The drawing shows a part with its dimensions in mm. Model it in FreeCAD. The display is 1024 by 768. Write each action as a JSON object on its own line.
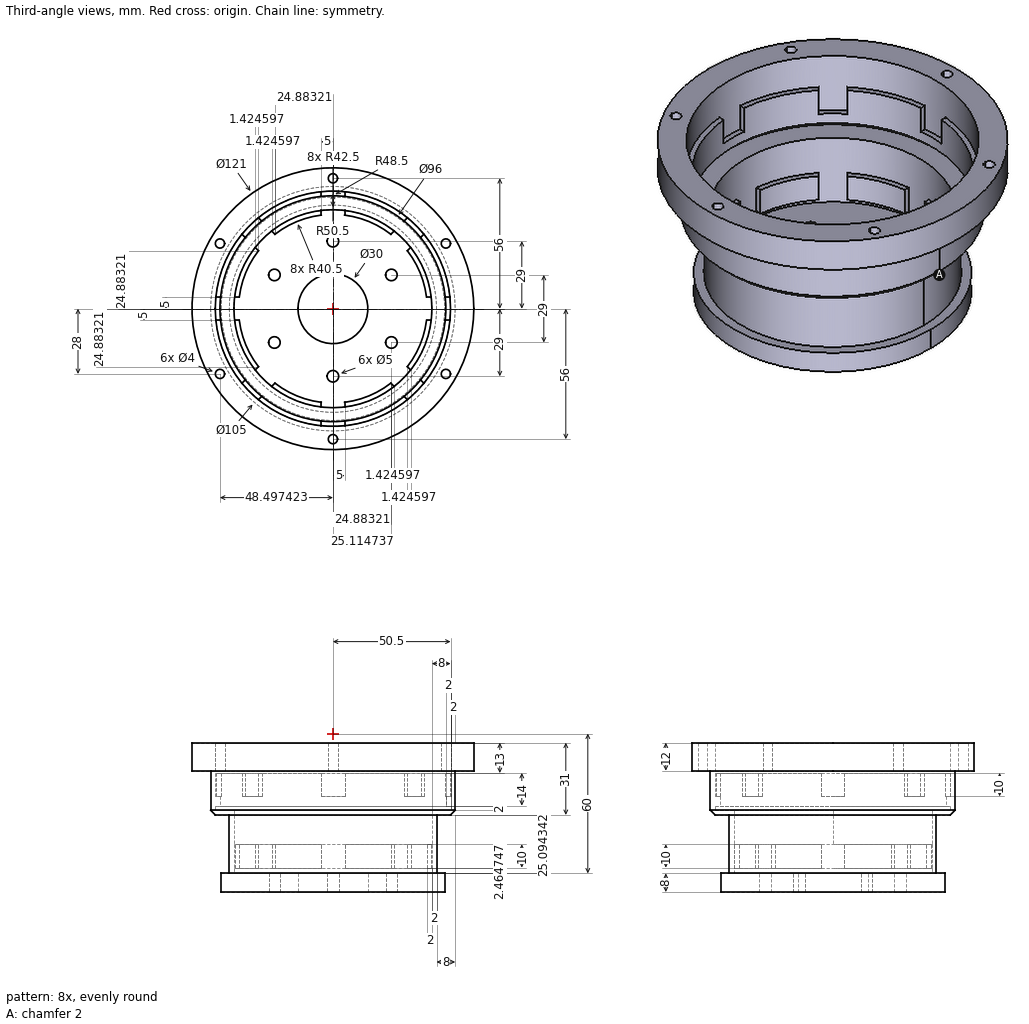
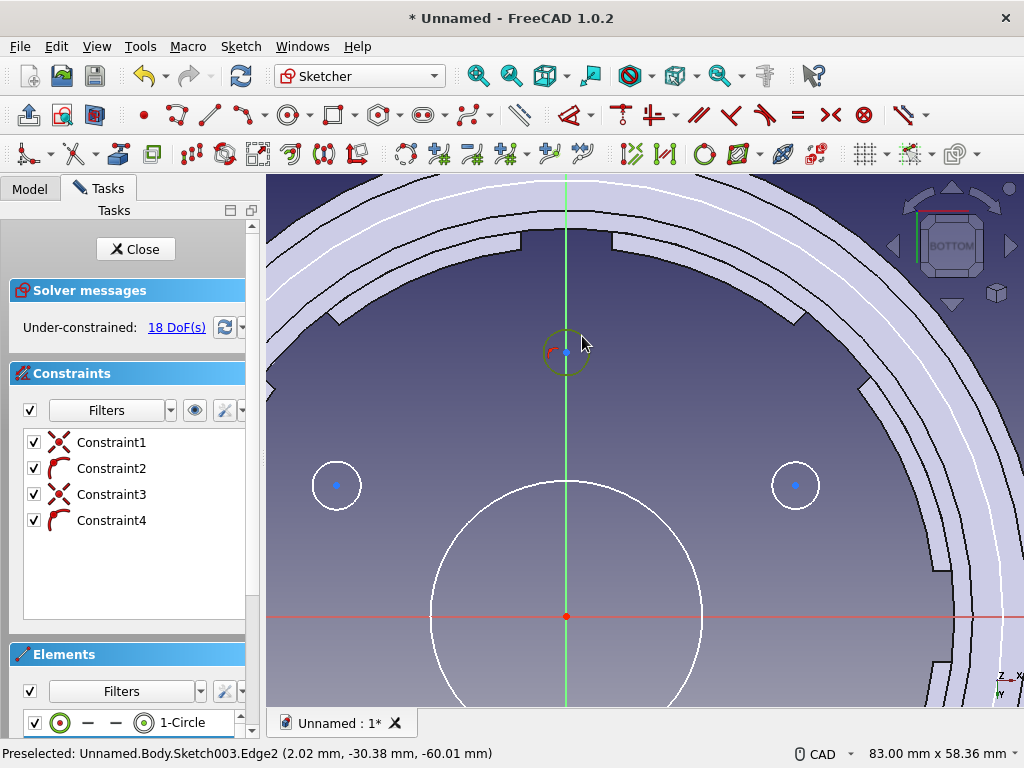
{"action": "left_click", "coordinate": [812, 469]}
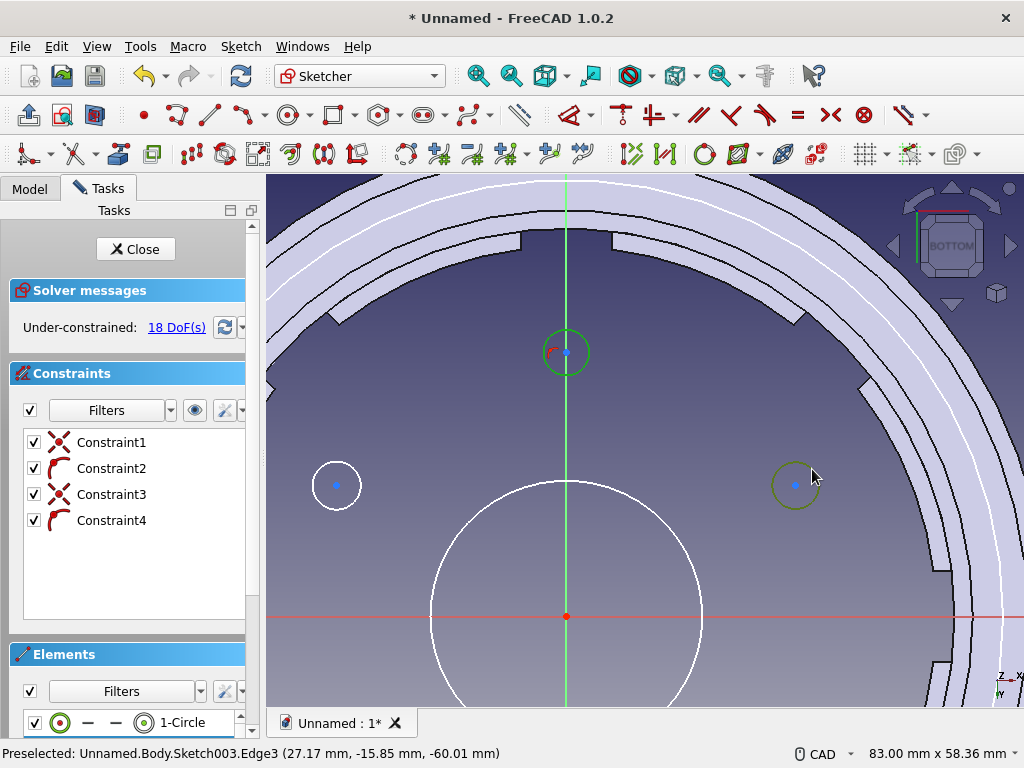
{"action": "left_click", "coordinate": [354, 469]}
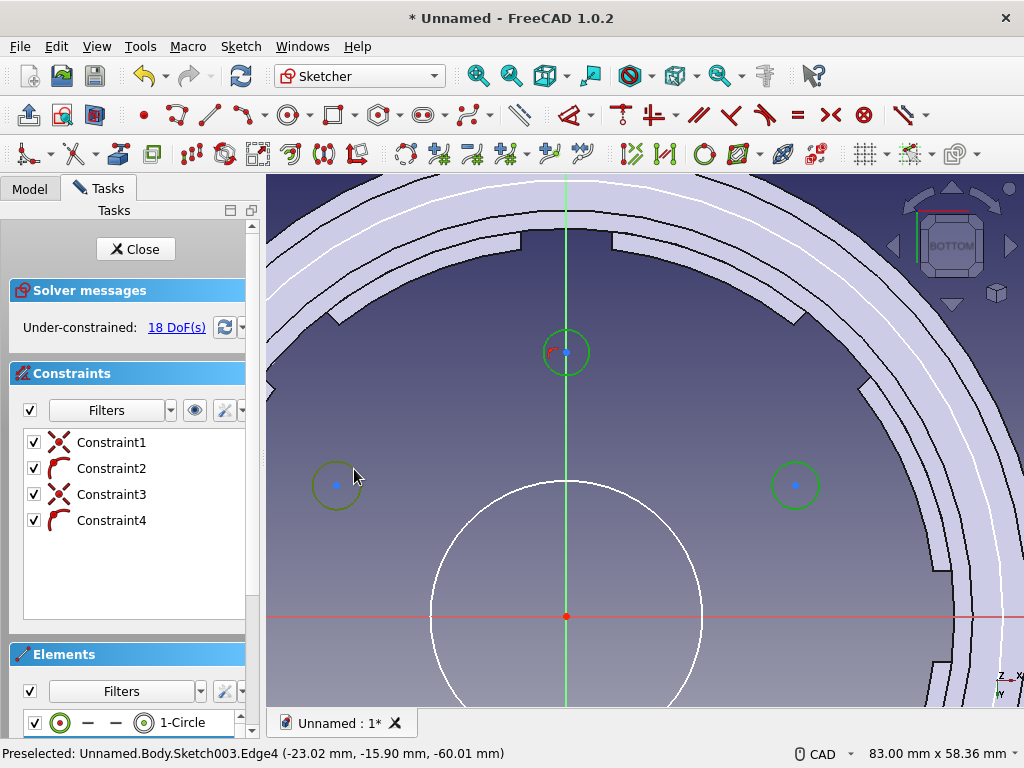
{"action": "scroll", "coordinate": [582, 338], "scroll_direction": "down", "scroll_amount": 5}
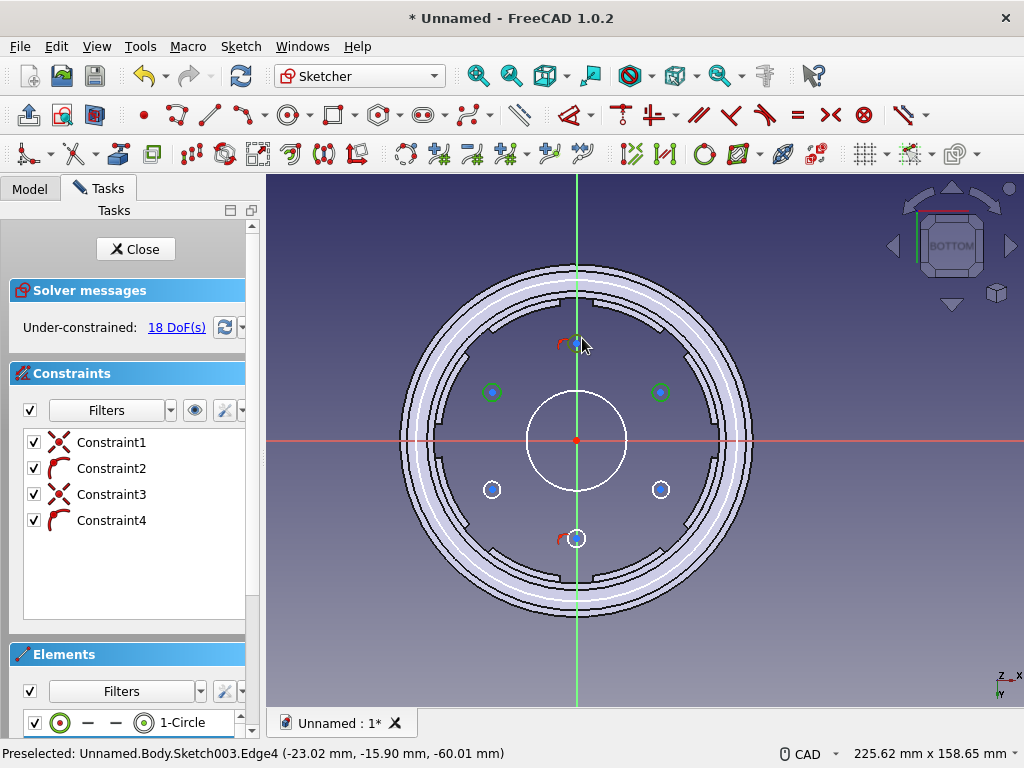
{"action": "scroll", "coordinate": [667, 484], "scroll_direction": "up", "scroll_amount": 3}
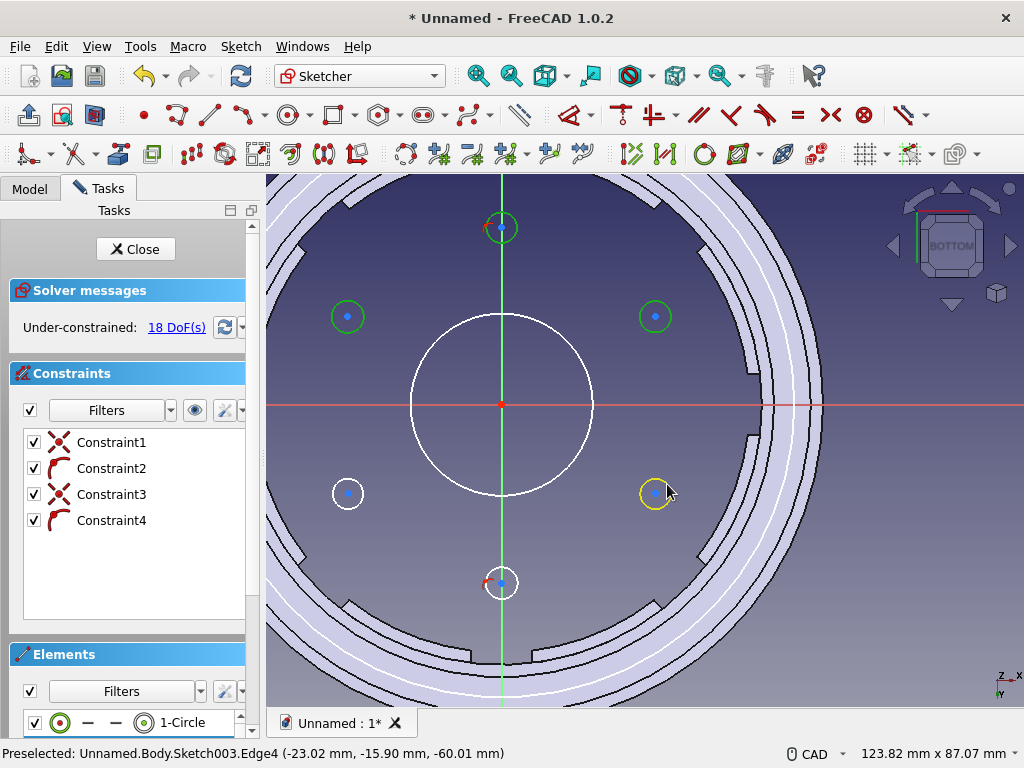
{"action": "left_click", "coordinate": [666, 483]}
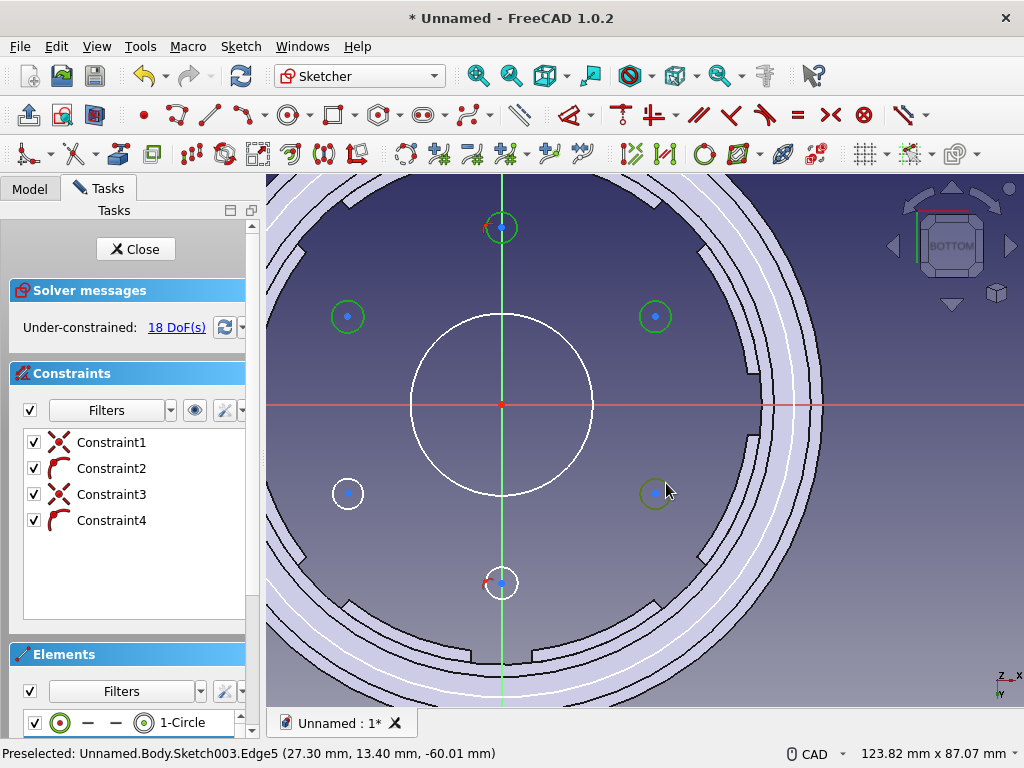
{"action": "scroll", "coordinate": [513, 572], "scroll_direction": "up", "scroll_amount": 2}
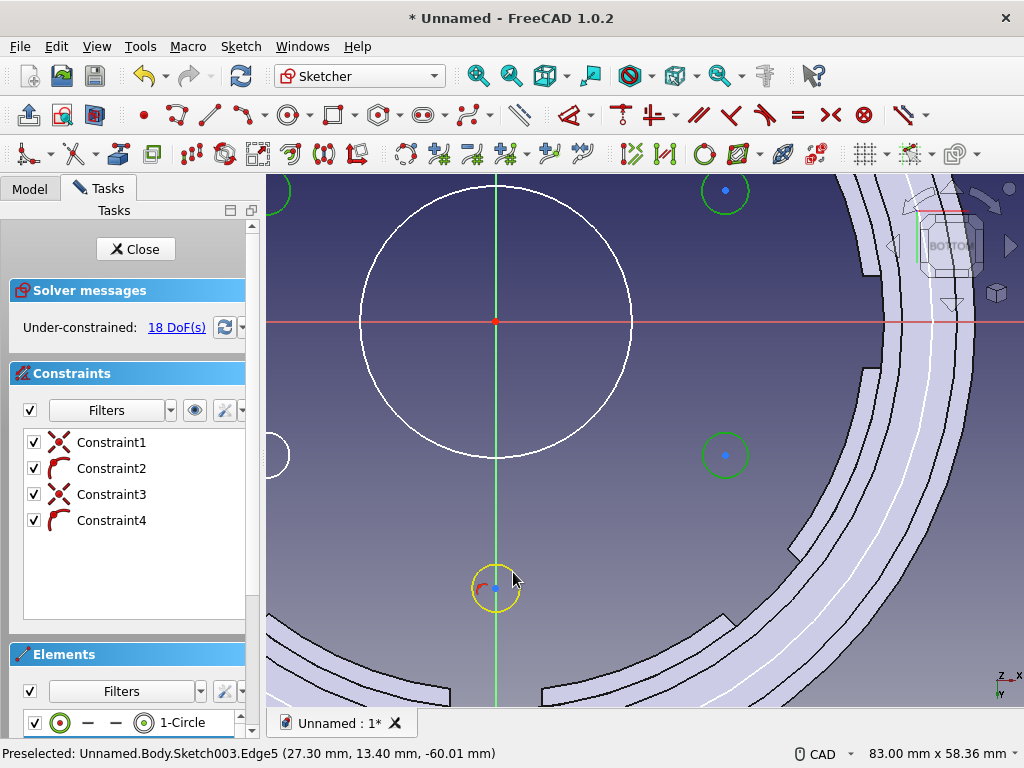
{"action": "left_click", "coordinate": [513, 571]}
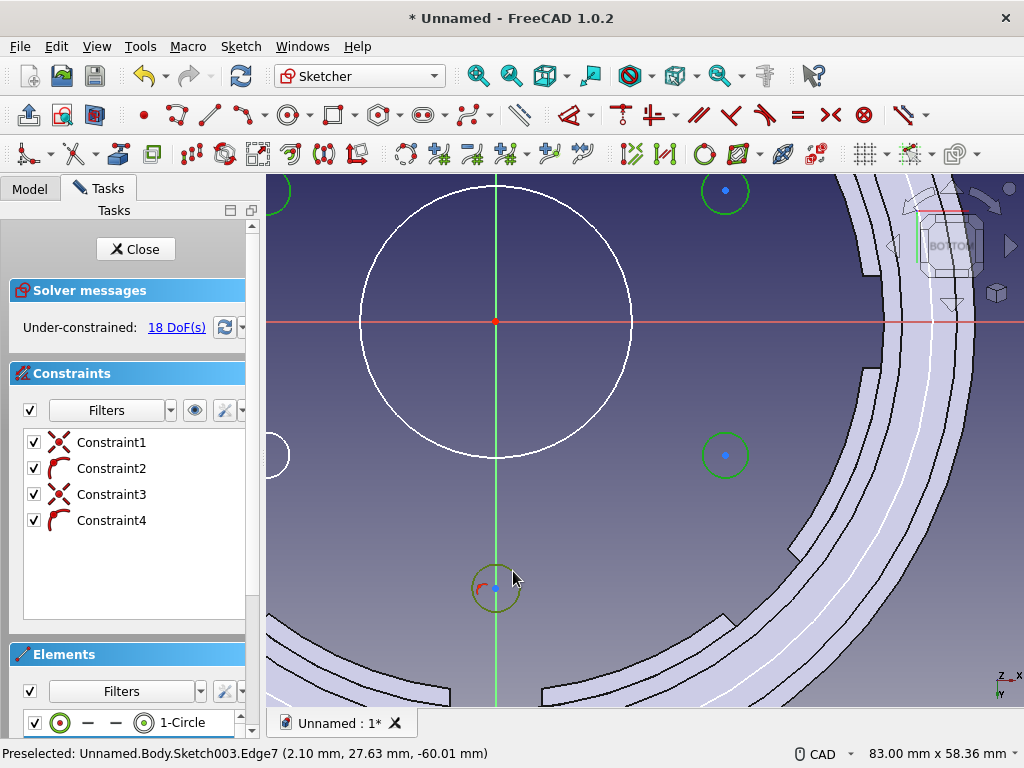
{"action": "scroll", "coordinate": [623, 509], "scroll_direction": "down", "scroll_amount": 5}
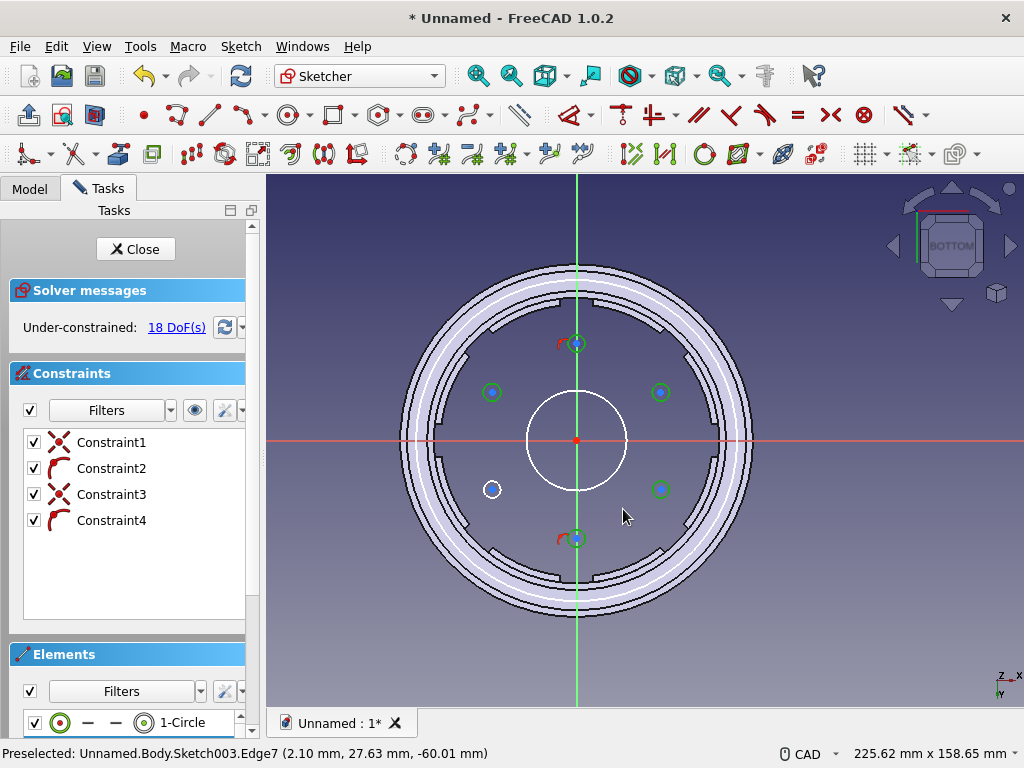
{"action": "scroll", "coordinate": [498, 484], "scroll_direction": "up", "scroll_amount": 3}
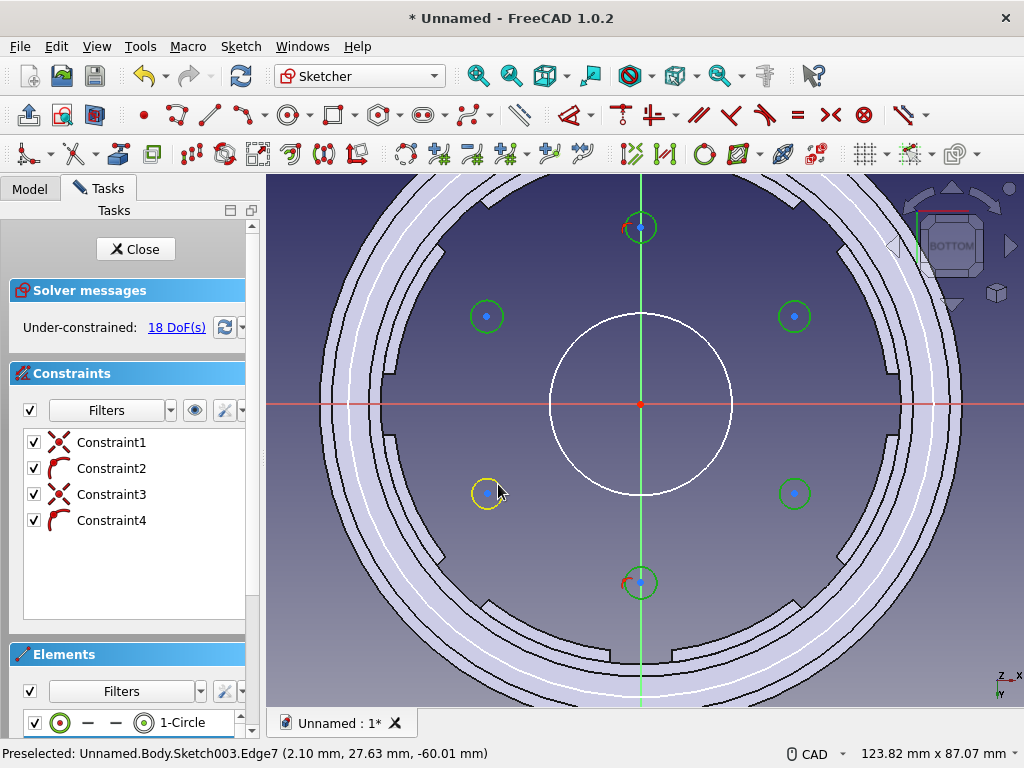
{"action": "left_click", "coordinate": [498, 483]}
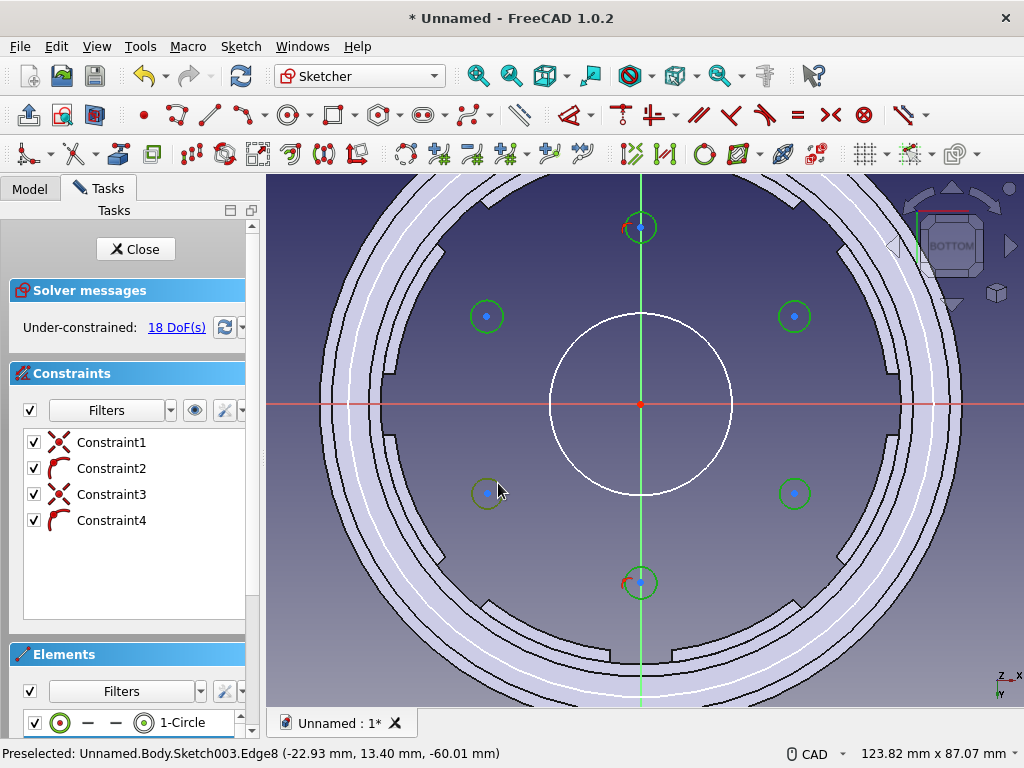
{"action": "key", "text": "e"}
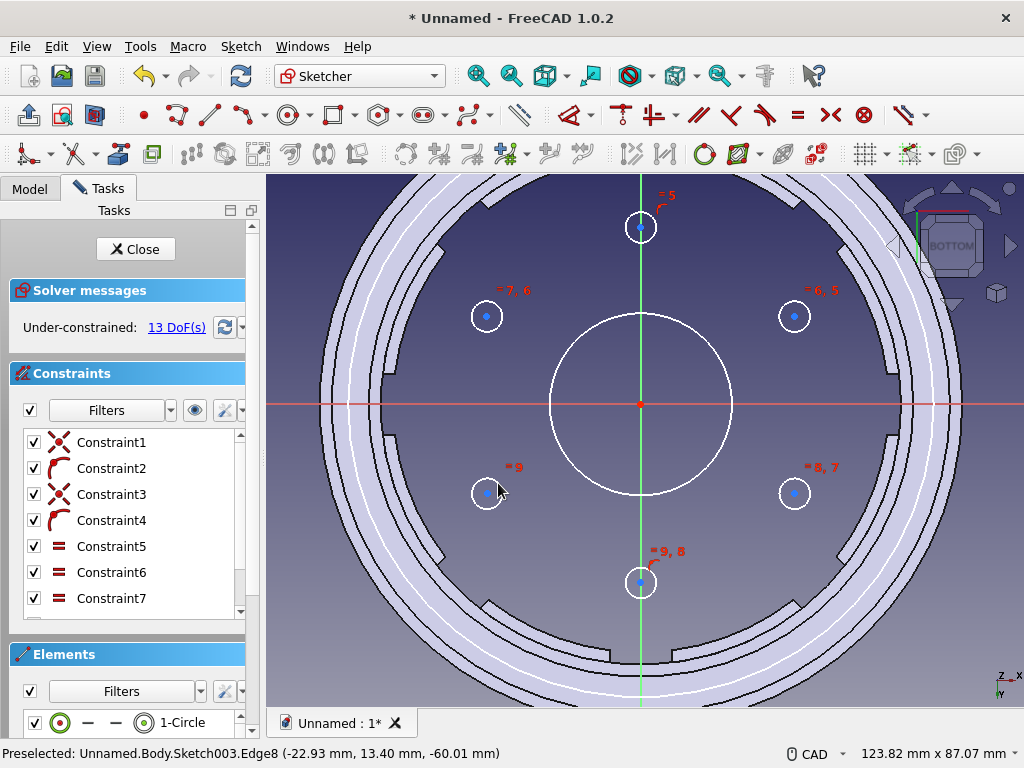
{"action": "left_click", "coordinate": [795, 317]}